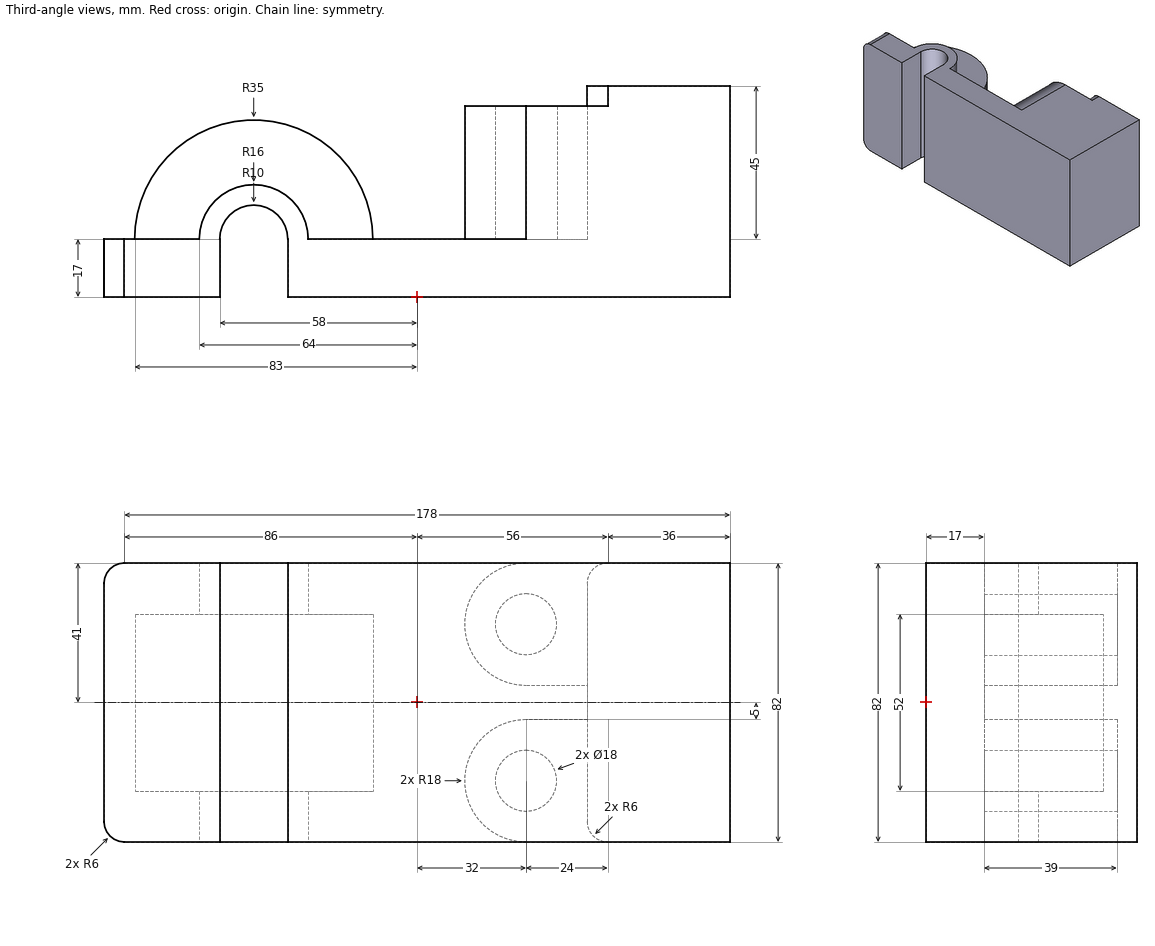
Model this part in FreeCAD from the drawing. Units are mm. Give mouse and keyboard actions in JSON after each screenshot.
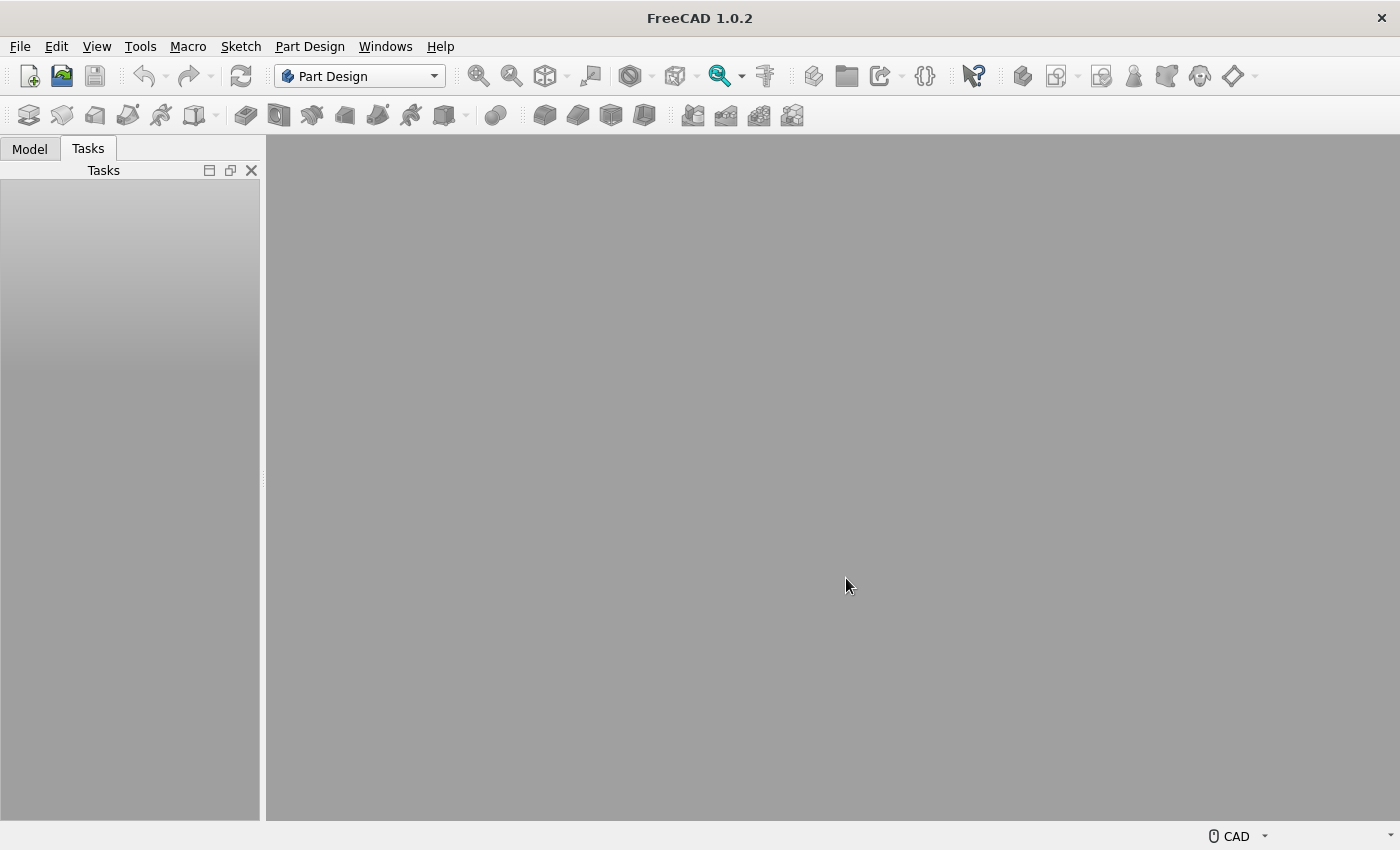
{"action": "left_click", "coordinate": [29, 76]}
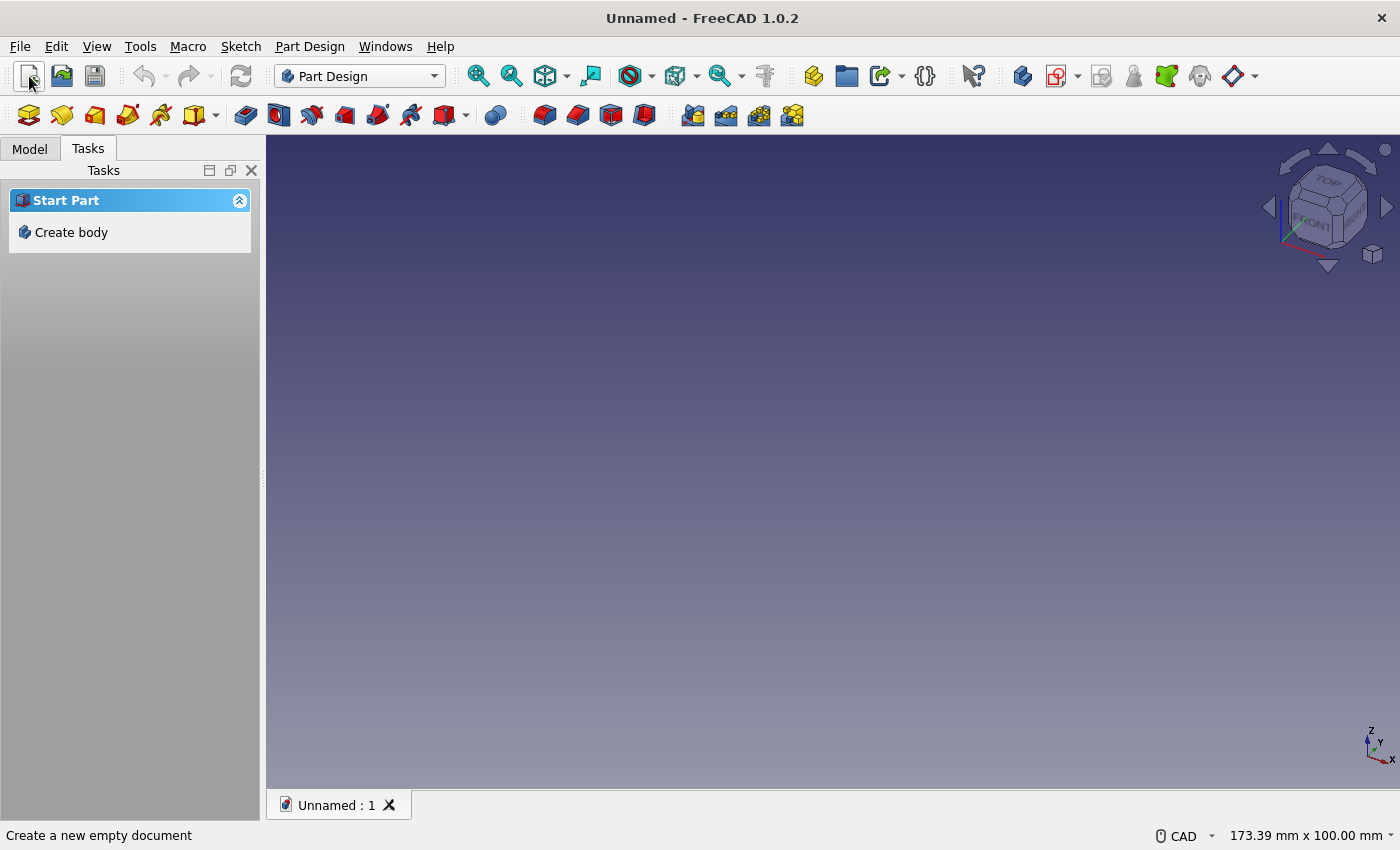
{"action": "left_click", "coordinate": [1056, 76]}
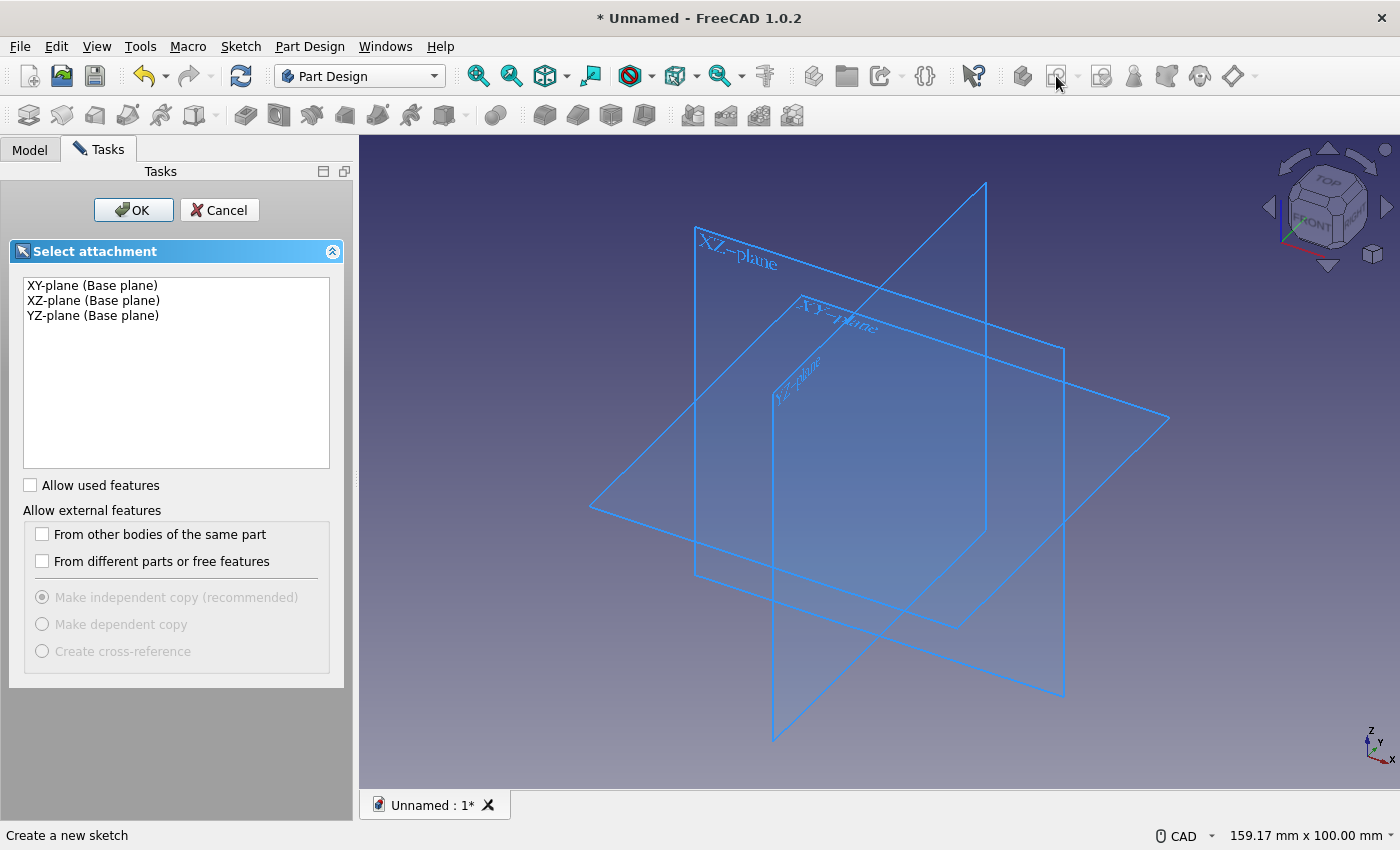
{"action": "left_click", "coordinate": [84, 300]}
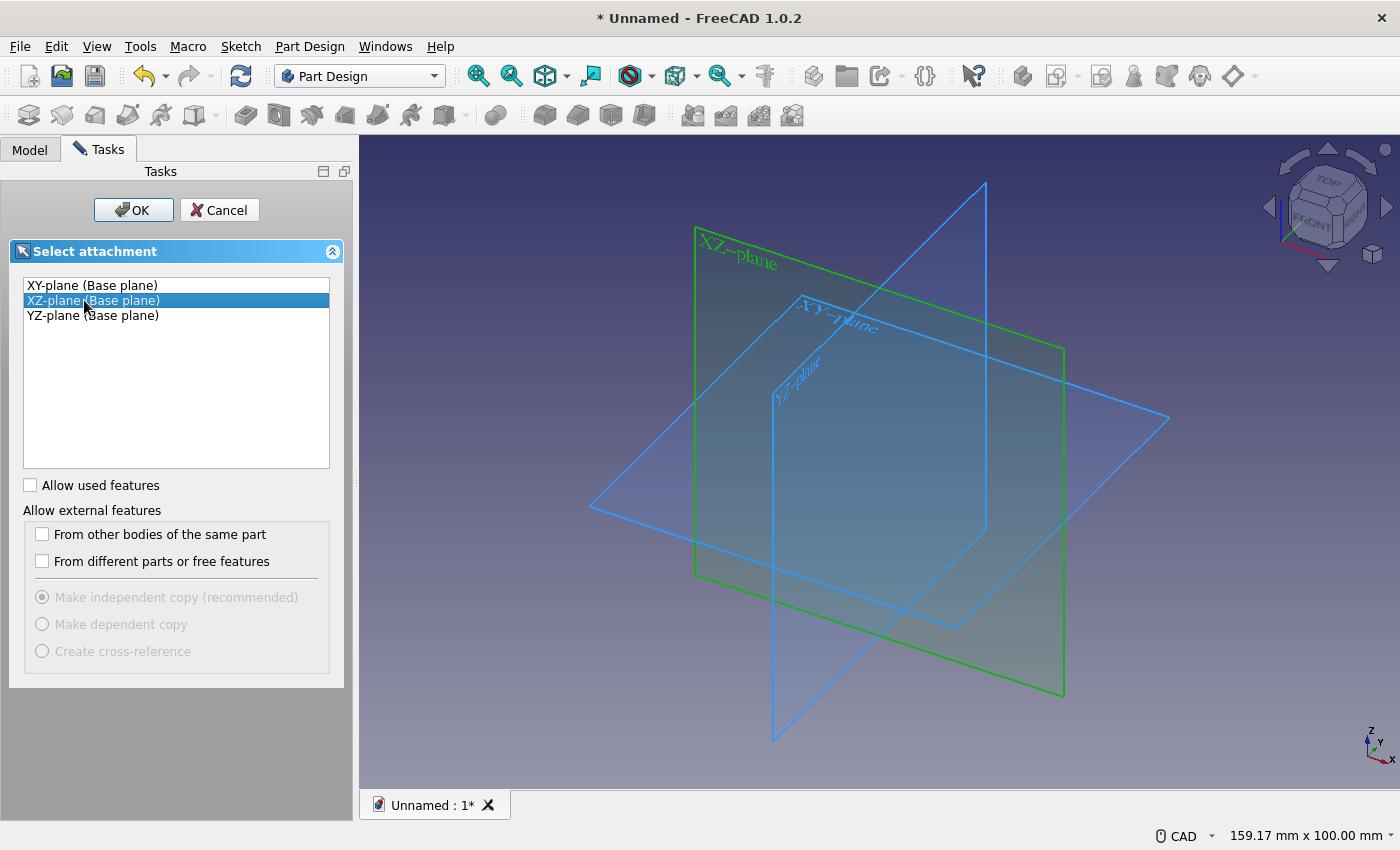
{"action": "left_click", "coordinate": [134, 210]}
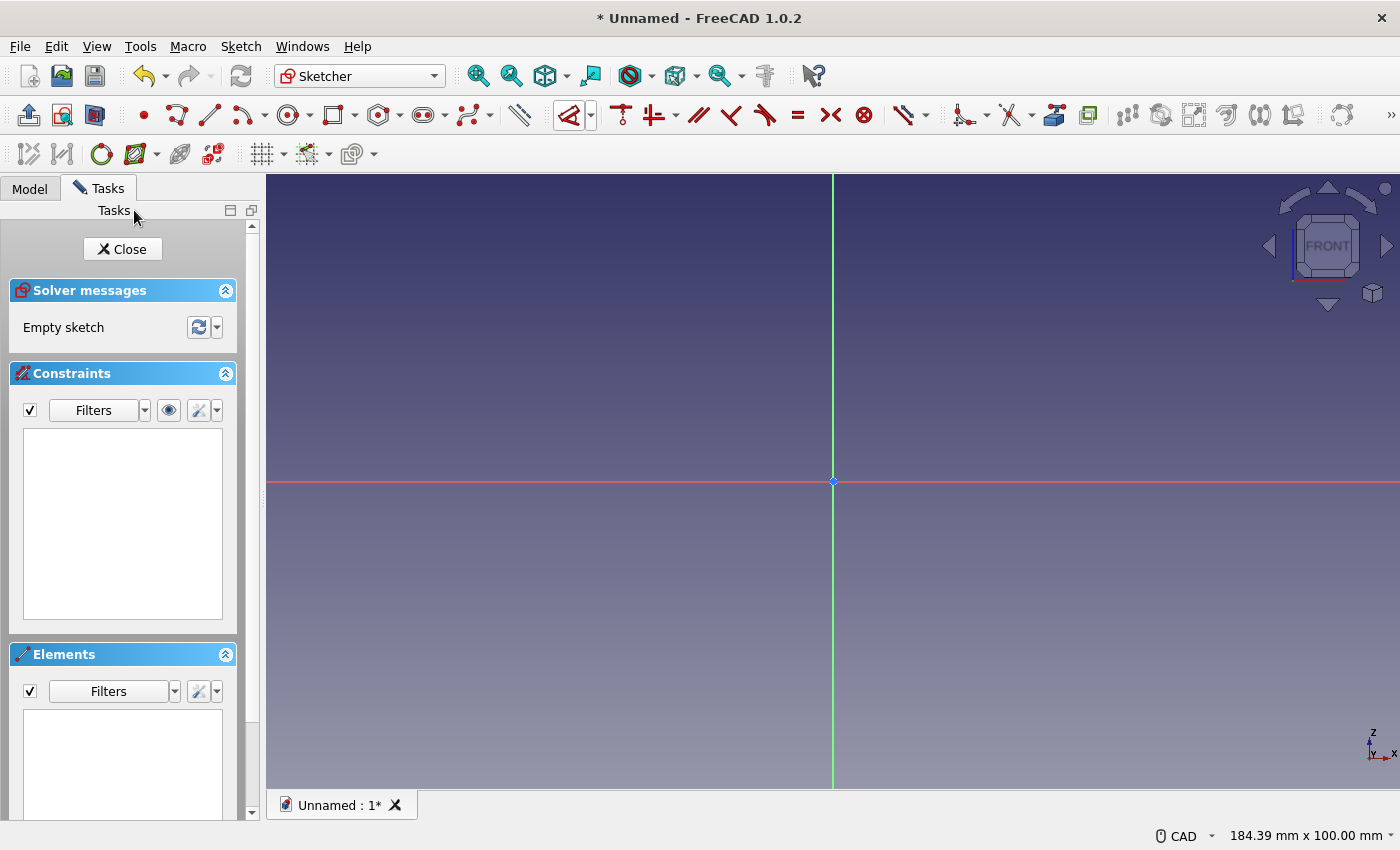
{"action": "scroll", "coordinate": [681, 482], "scroll_direction": "down", "scroll_amount": 3}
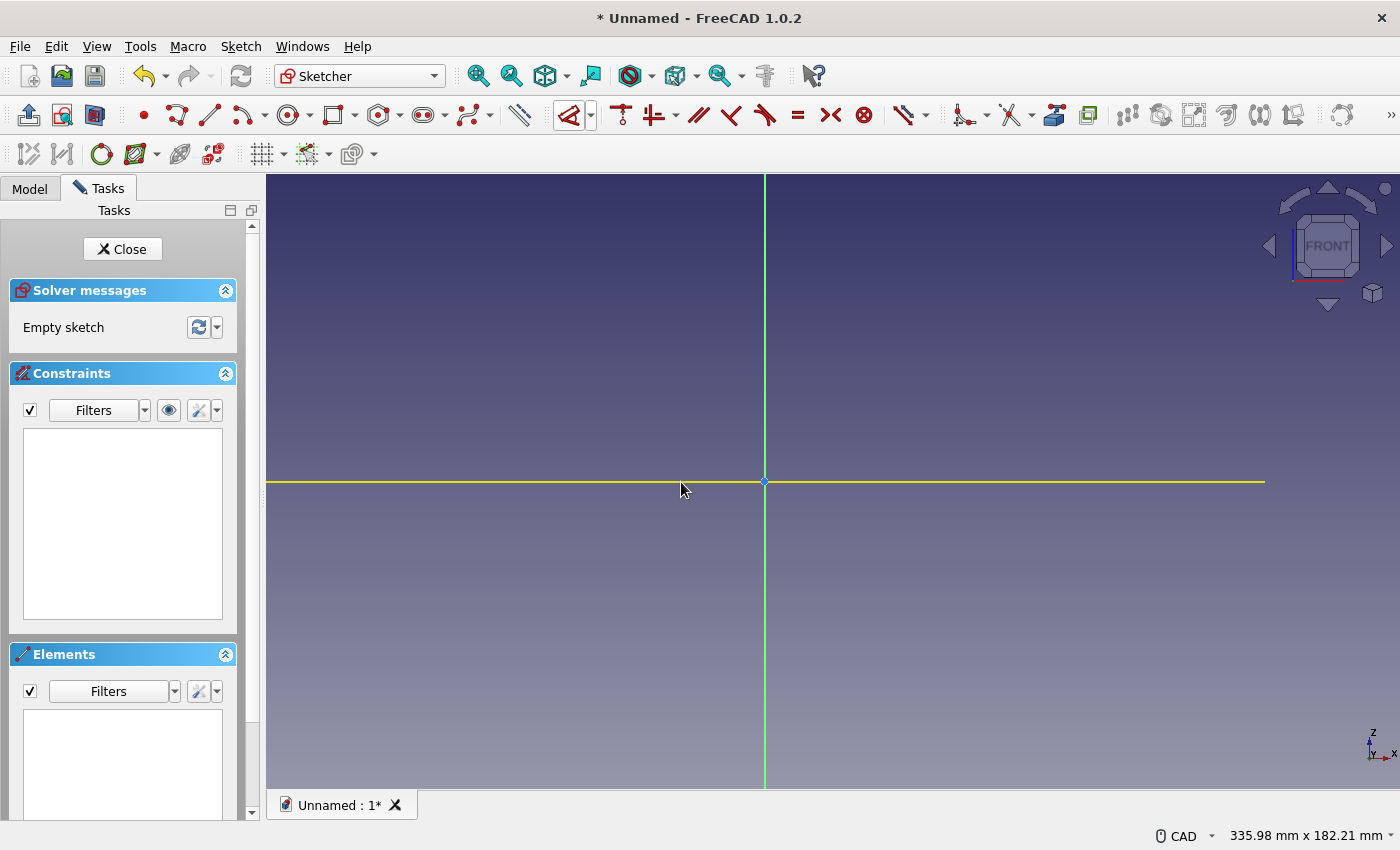
{"action": "left_click", "coordinate": [177, 116]}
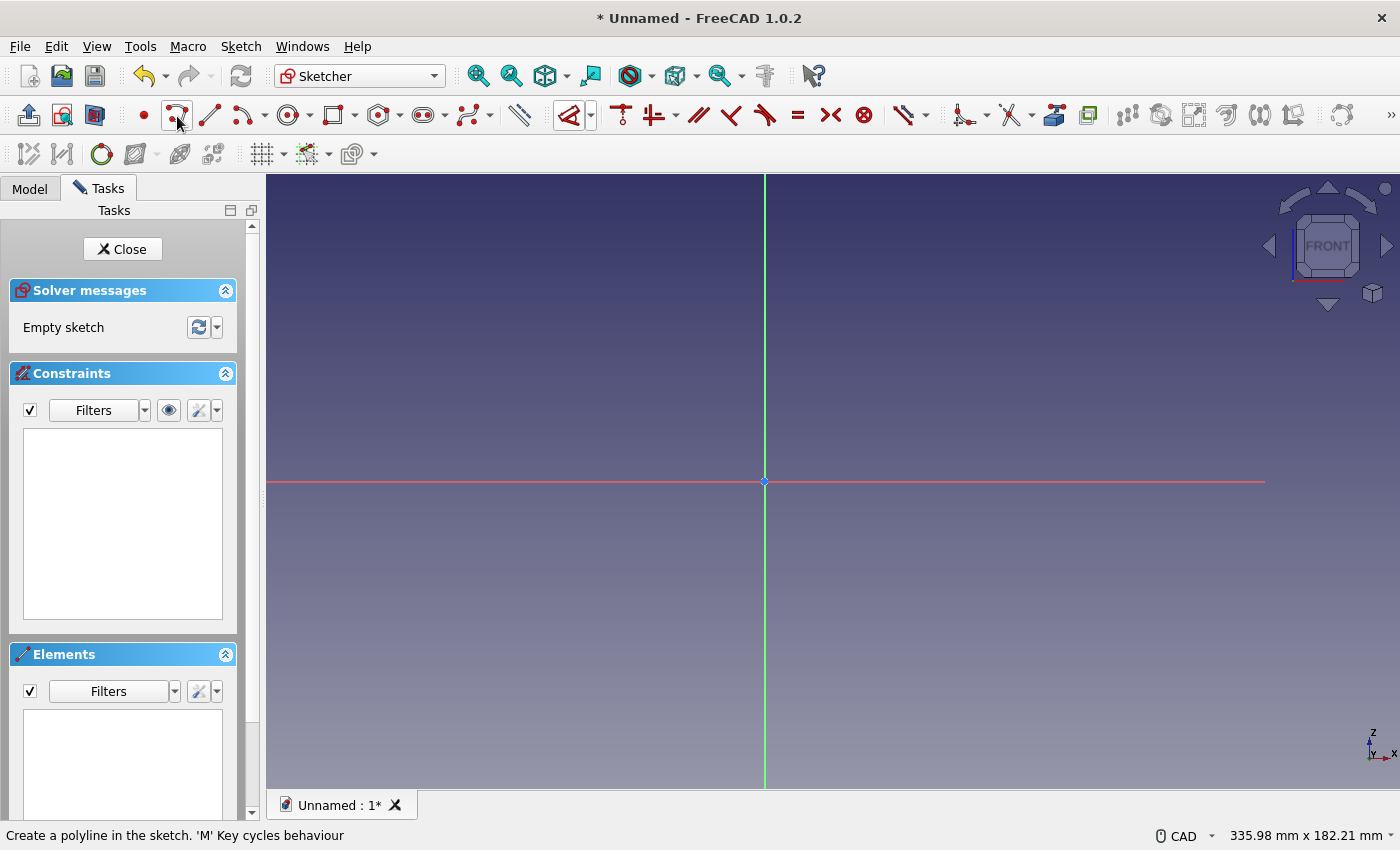
{"action": "left_click", "coordinate": [474, 344]}
{"action": "left_click", "coordinate": [1075, 344]}
{"action": "left_click", "coordinate": [1075, 620]}
{"action": "left_click", "coordinate": [474, 620]}
{"action": "right_click", "coordinate": [474, 620]}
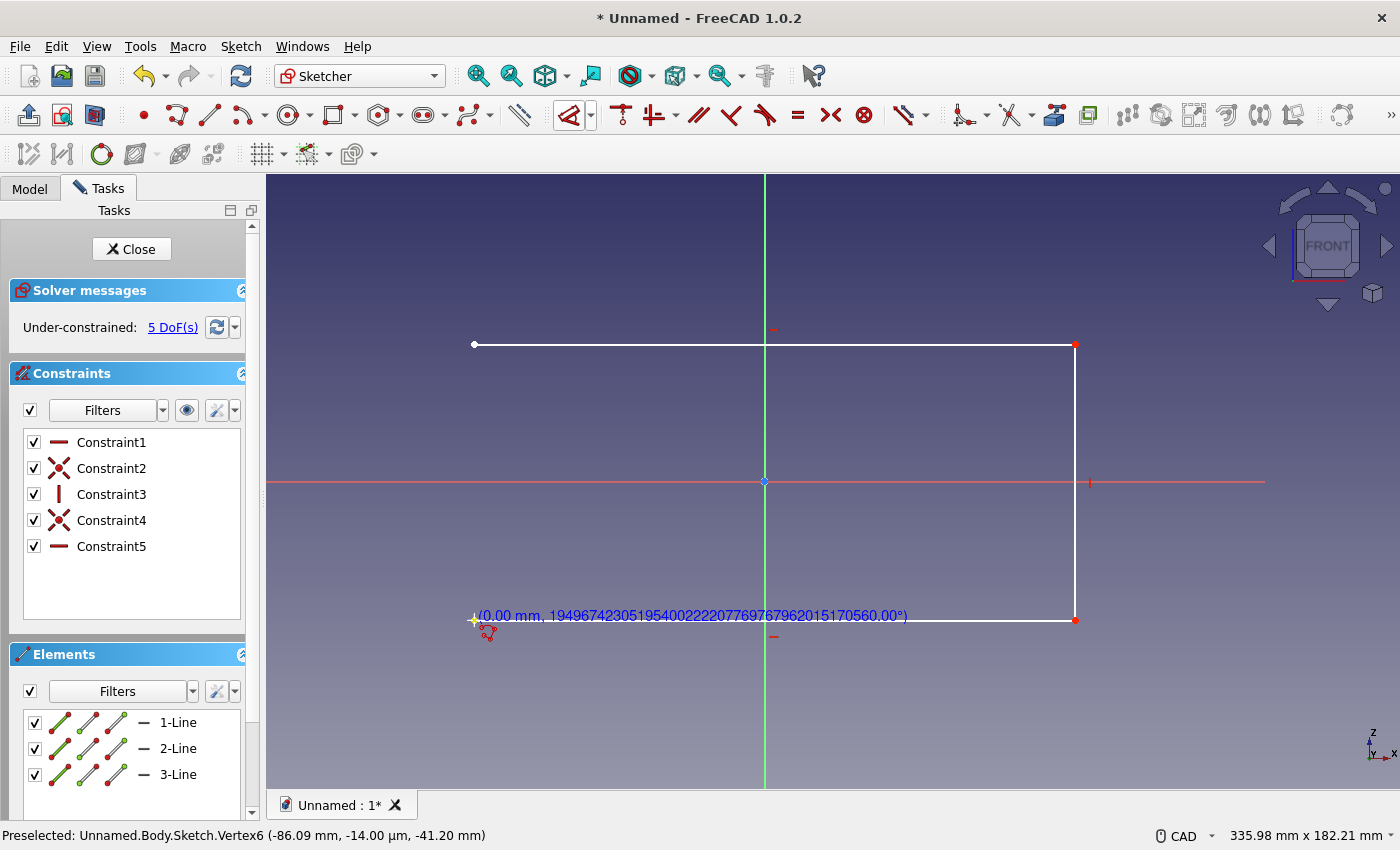
{"action": "left_click", "coordinate": [210, 116]}